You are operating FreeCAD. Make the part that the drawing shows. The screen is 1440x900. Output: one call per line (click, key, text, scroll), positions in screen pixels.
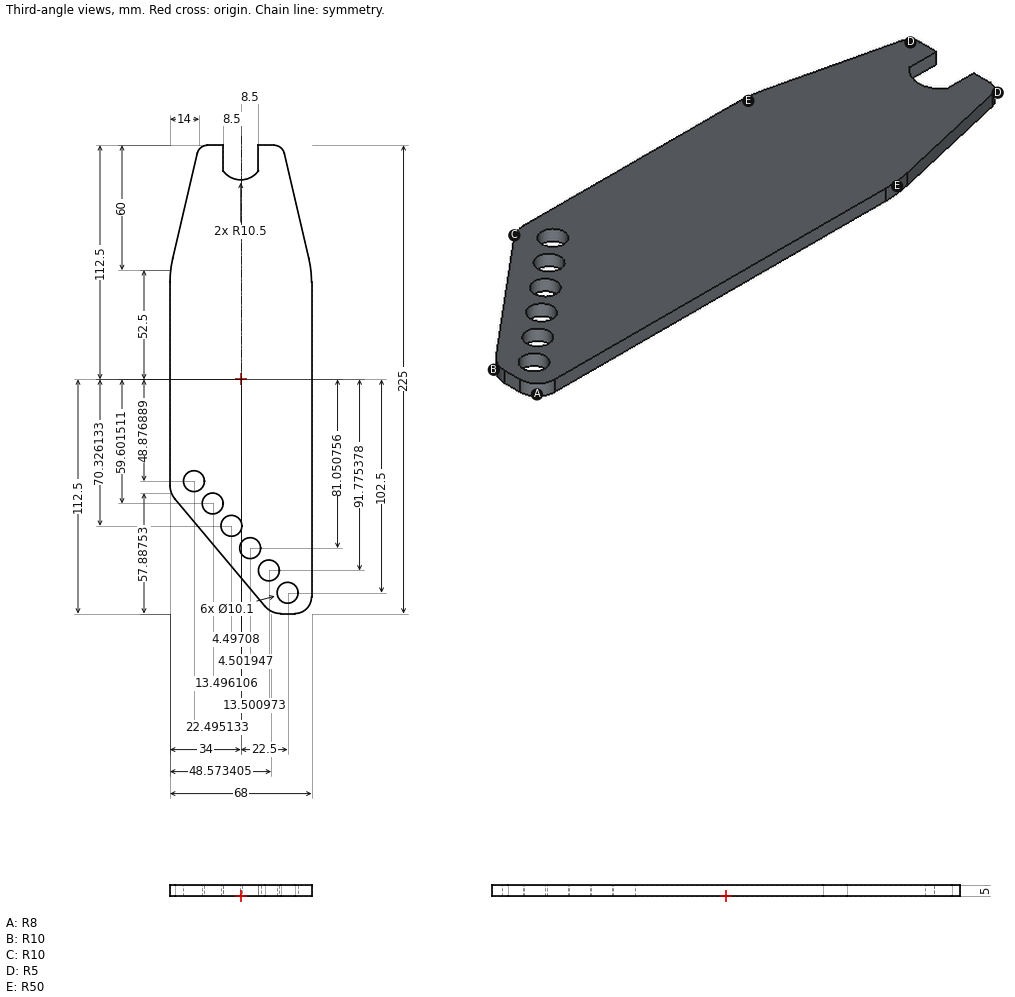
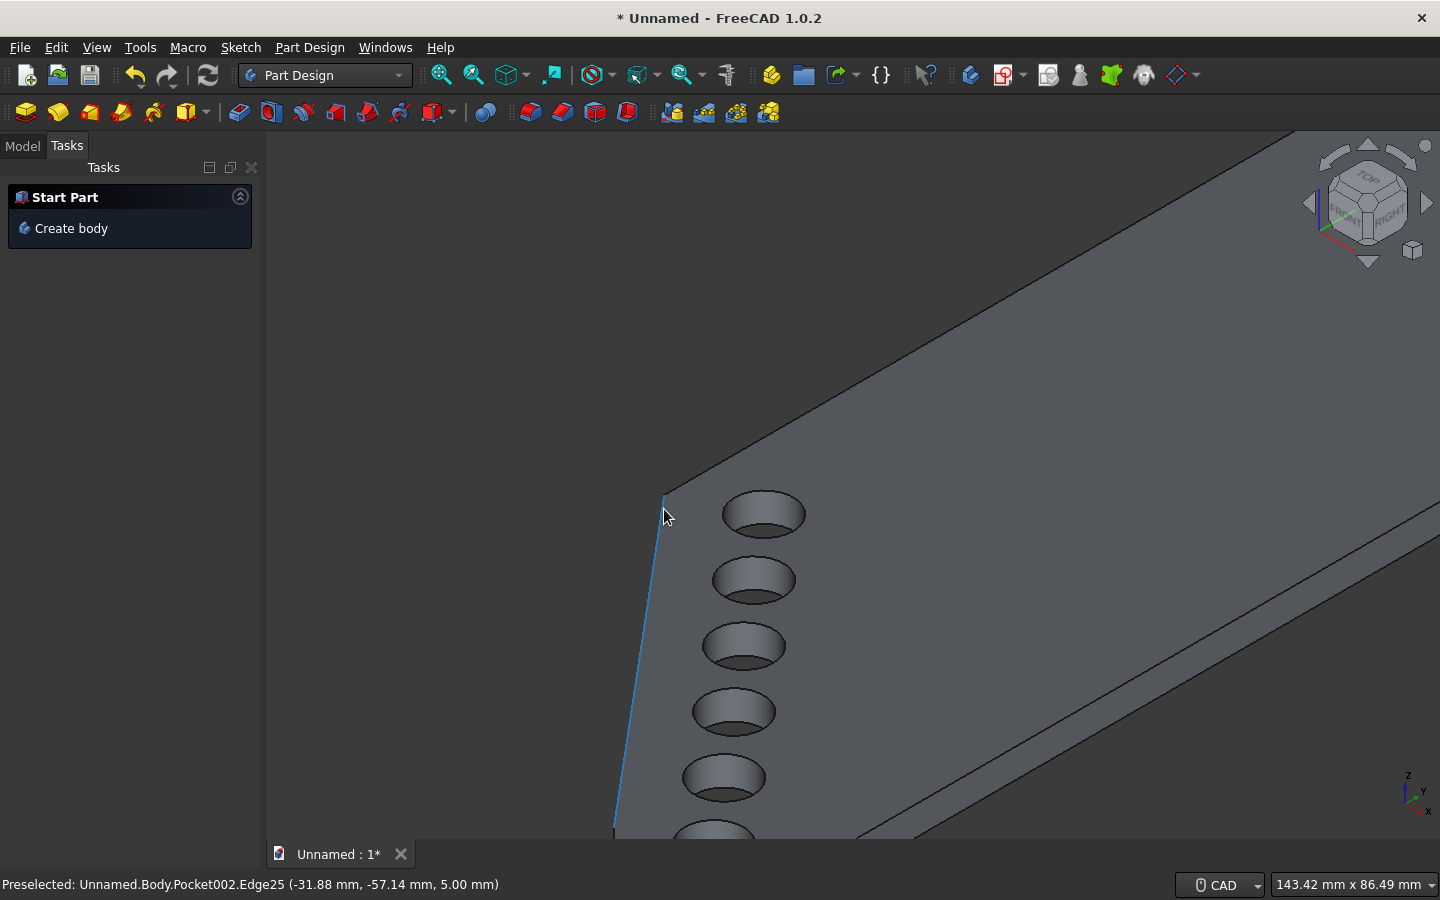
click(442, 76)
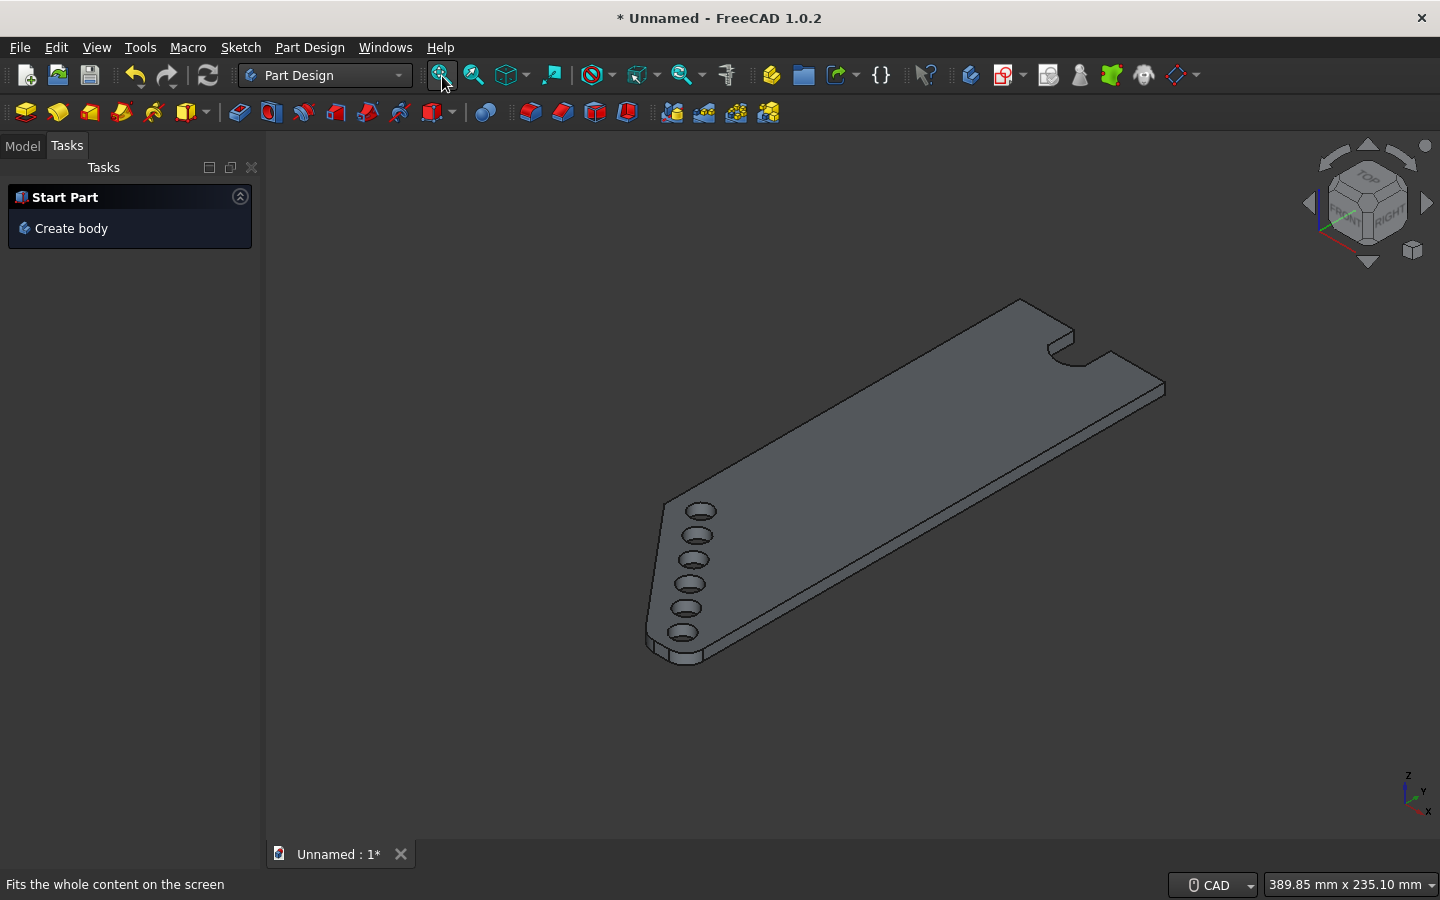
key(2)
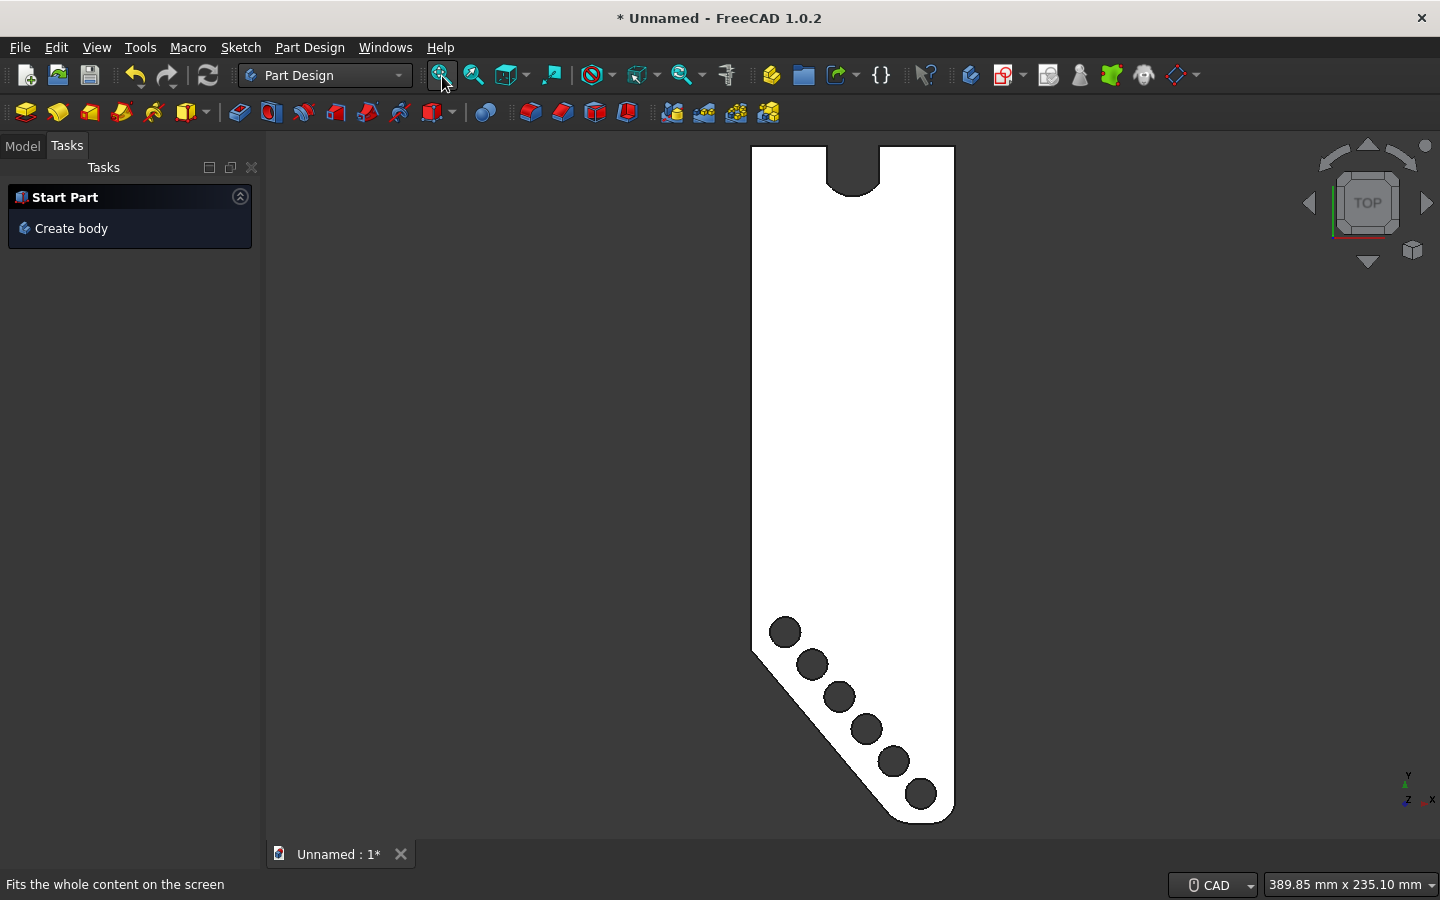
scroll(751, 648, up, 5)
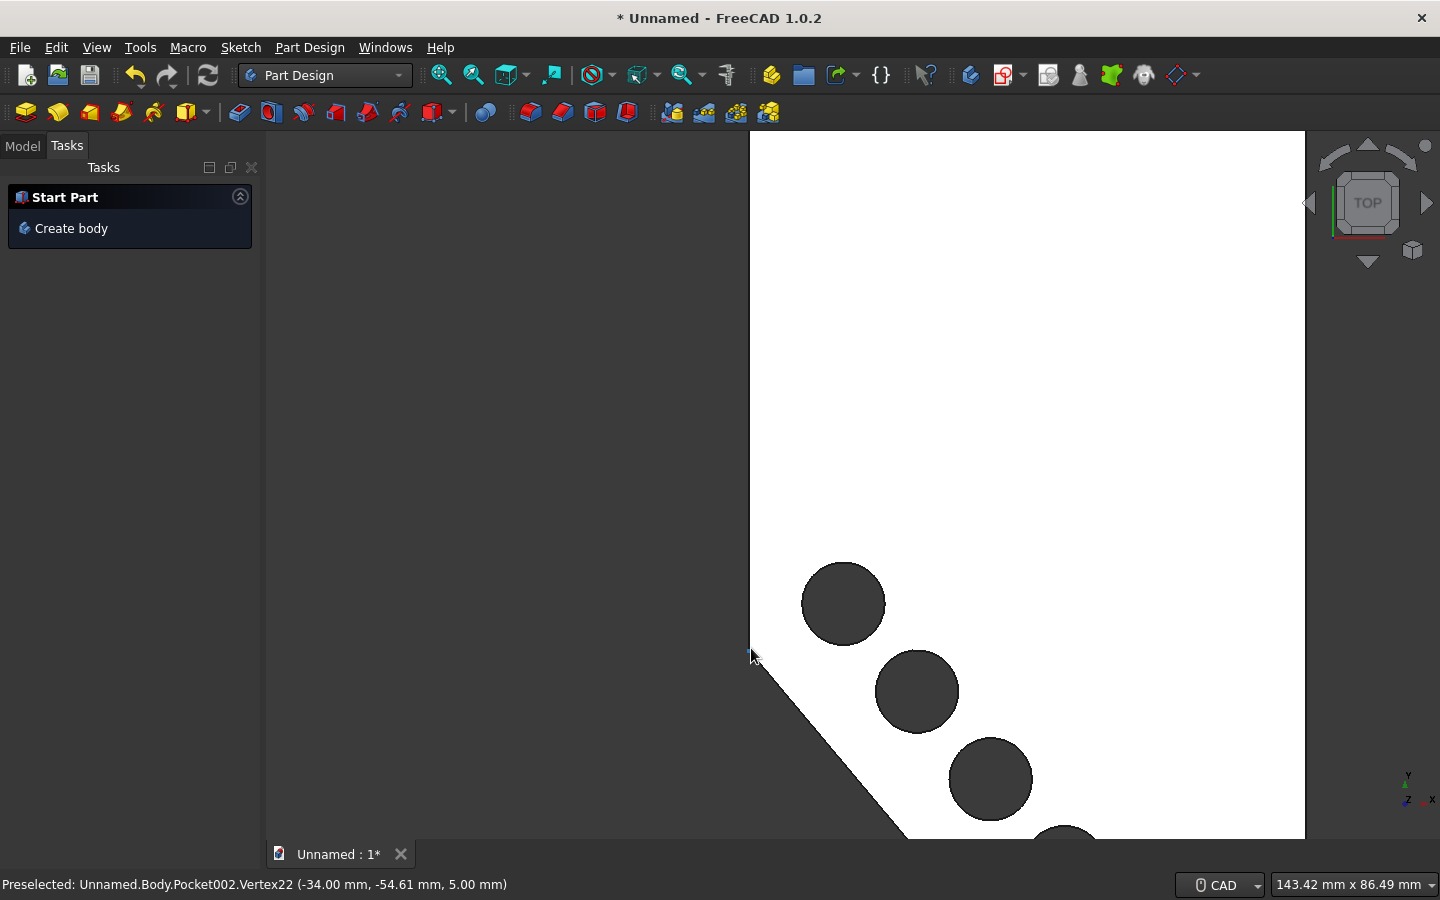
key(v)
key(f)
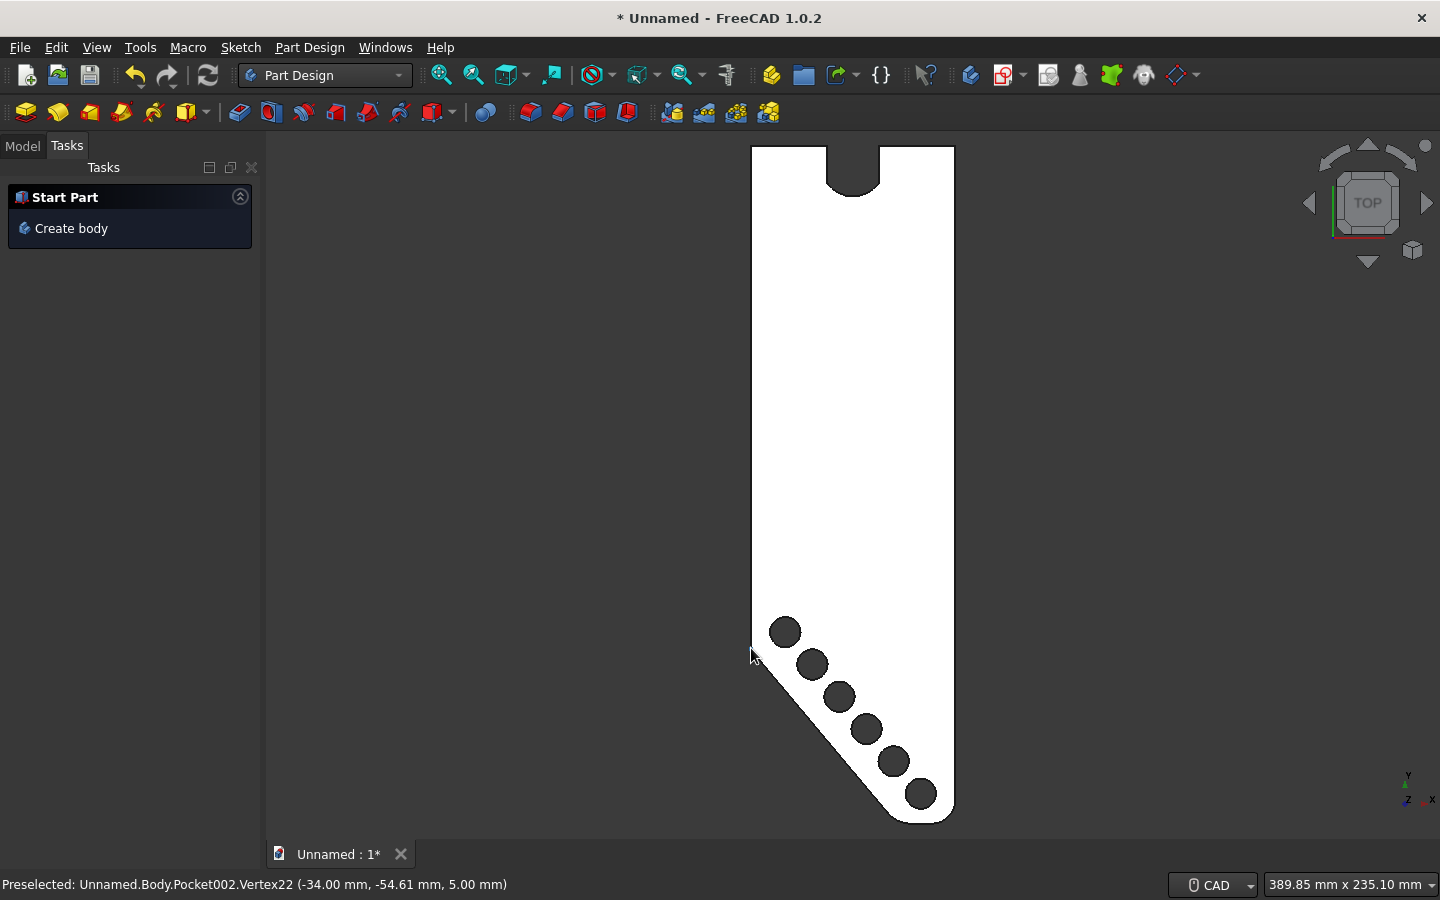
key(0)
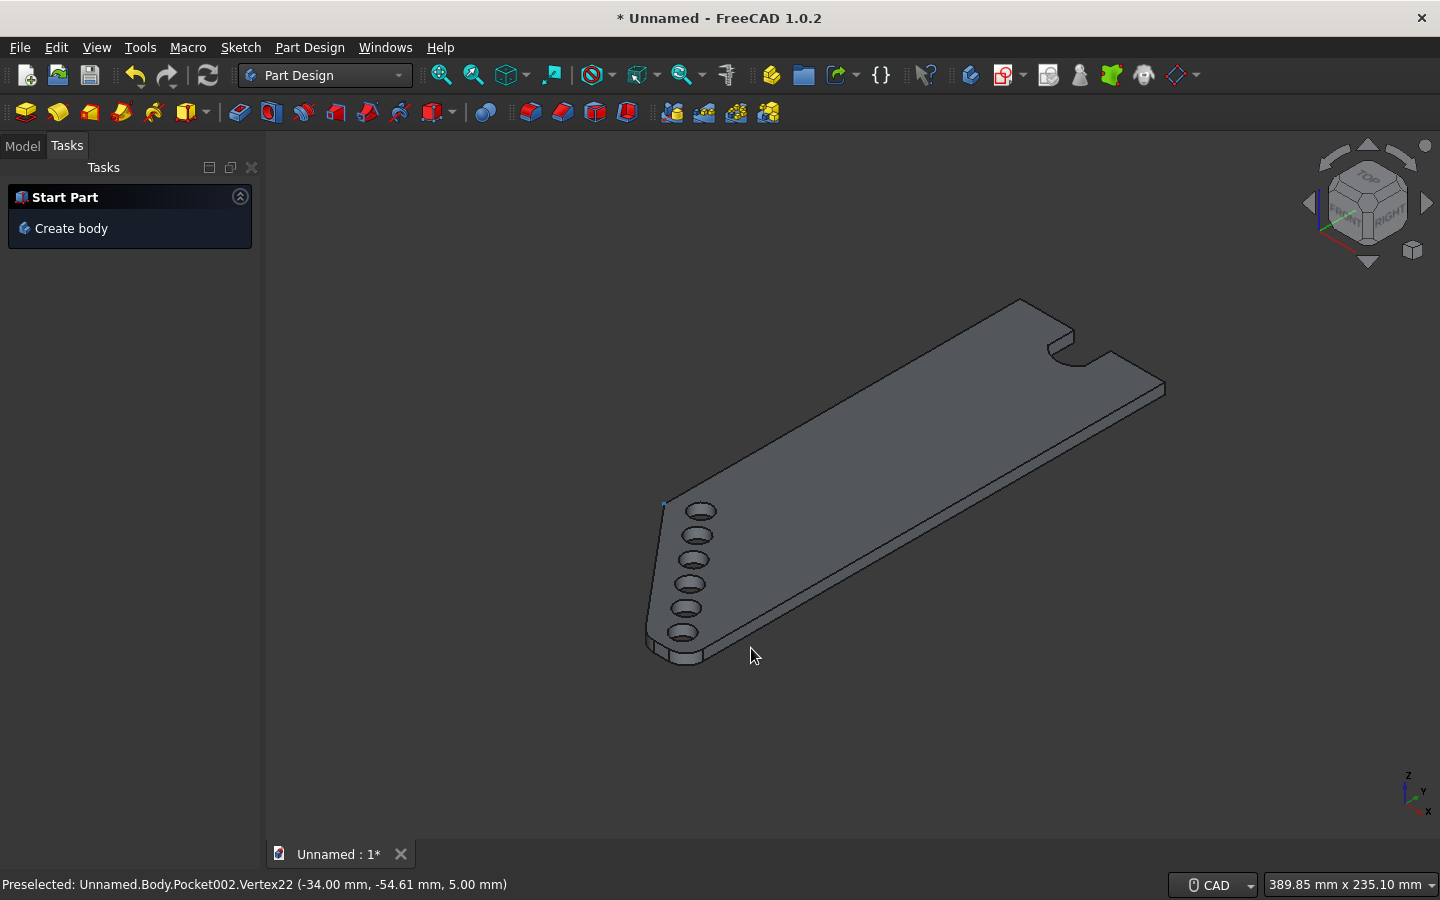
scroll(664, 509, up, 5)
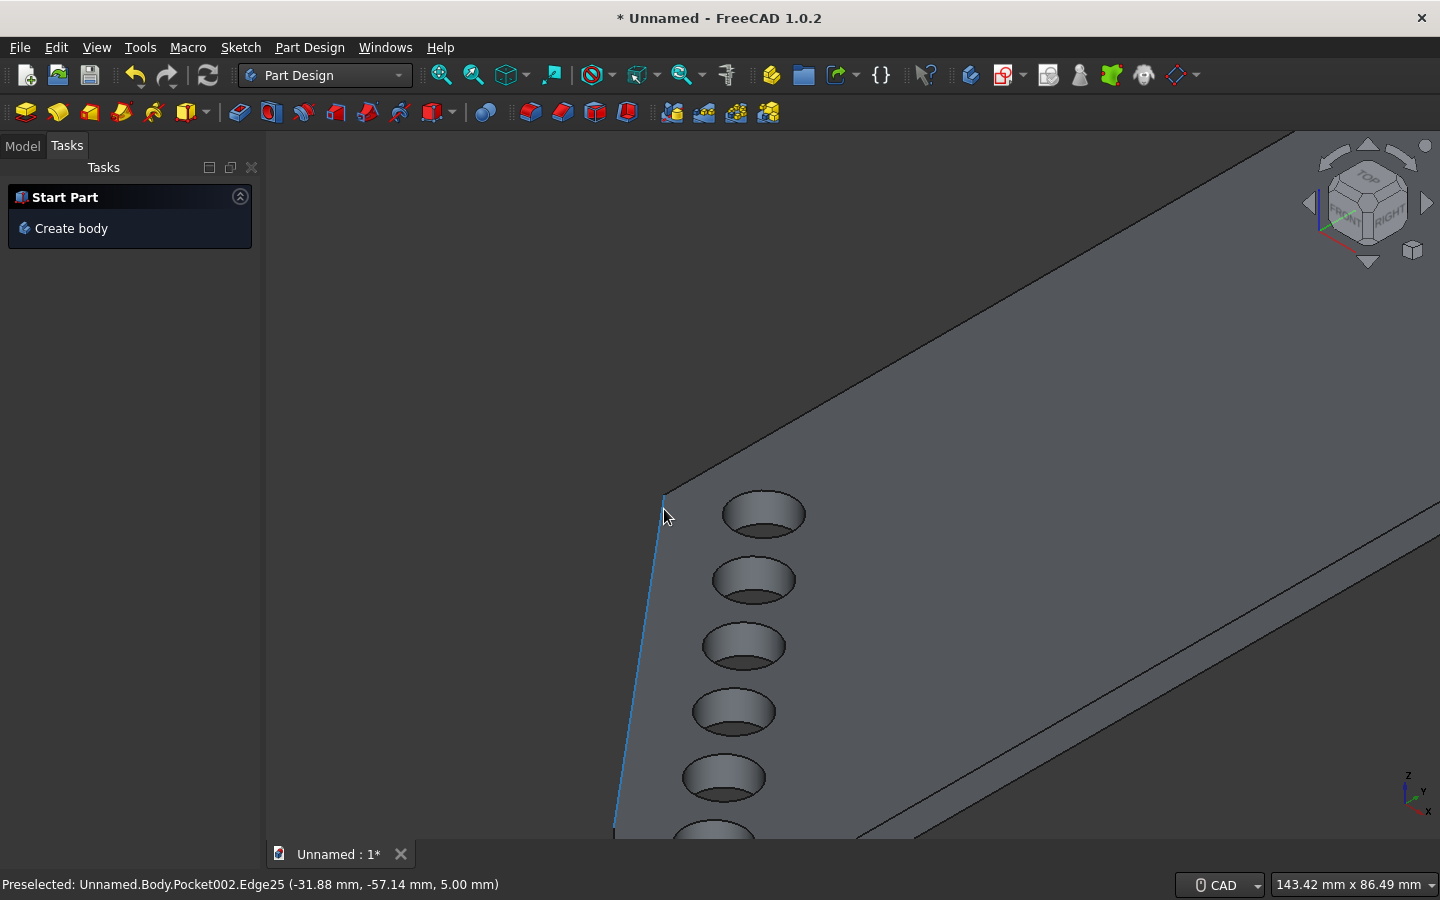
click(442, 76)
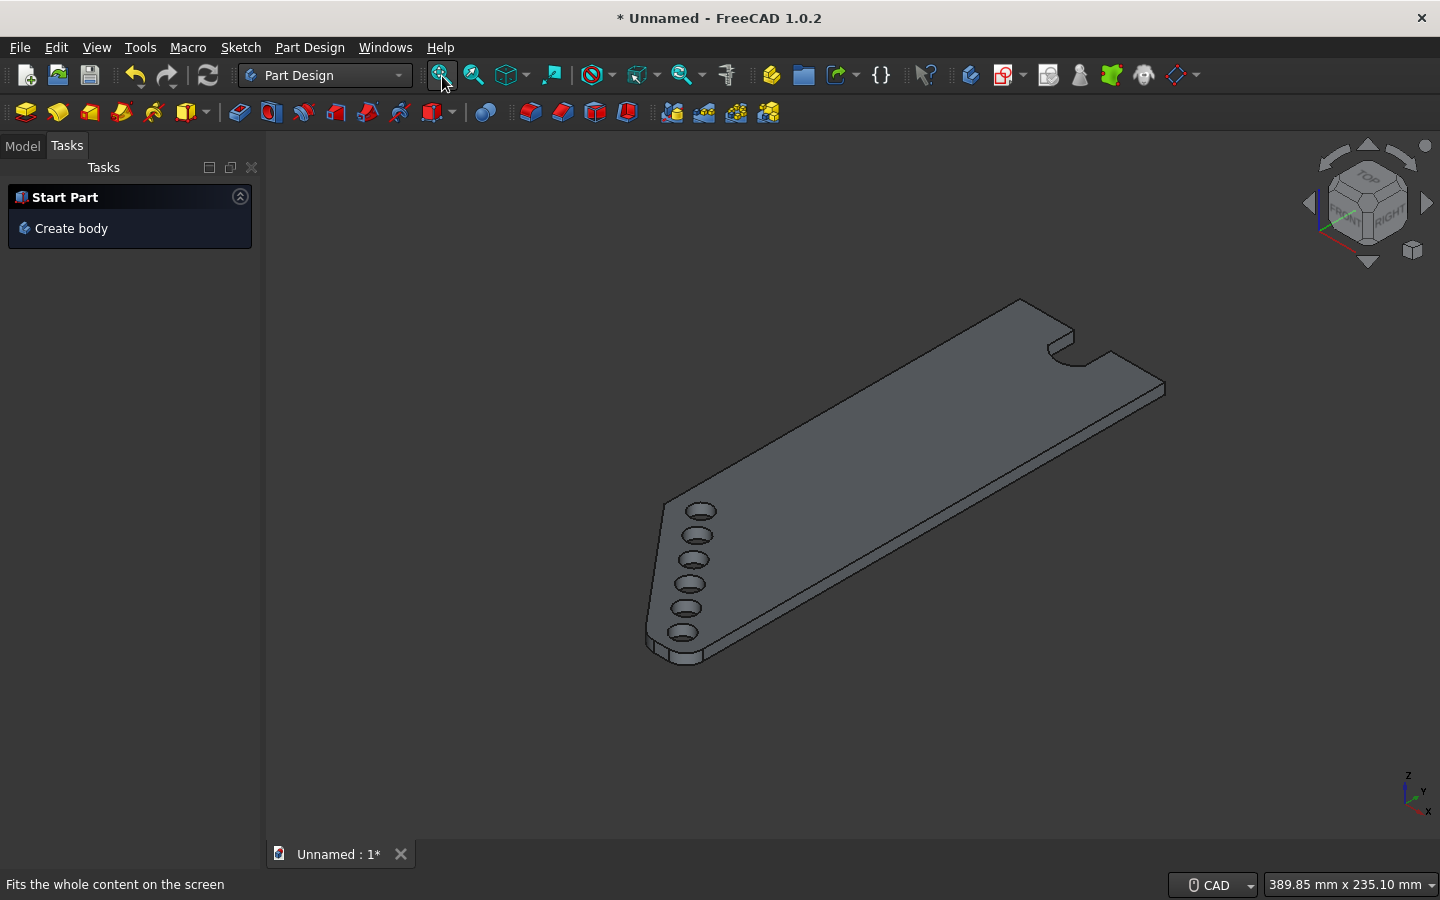
key(1)